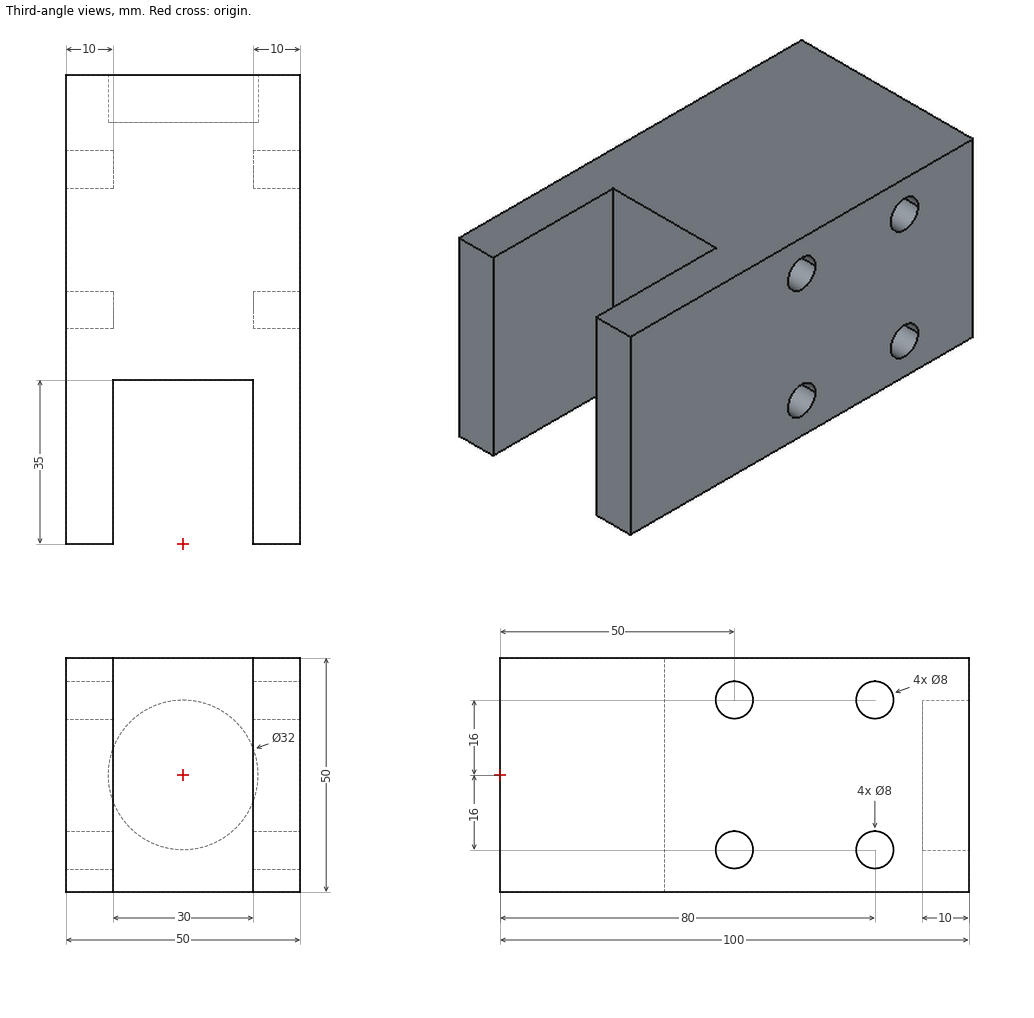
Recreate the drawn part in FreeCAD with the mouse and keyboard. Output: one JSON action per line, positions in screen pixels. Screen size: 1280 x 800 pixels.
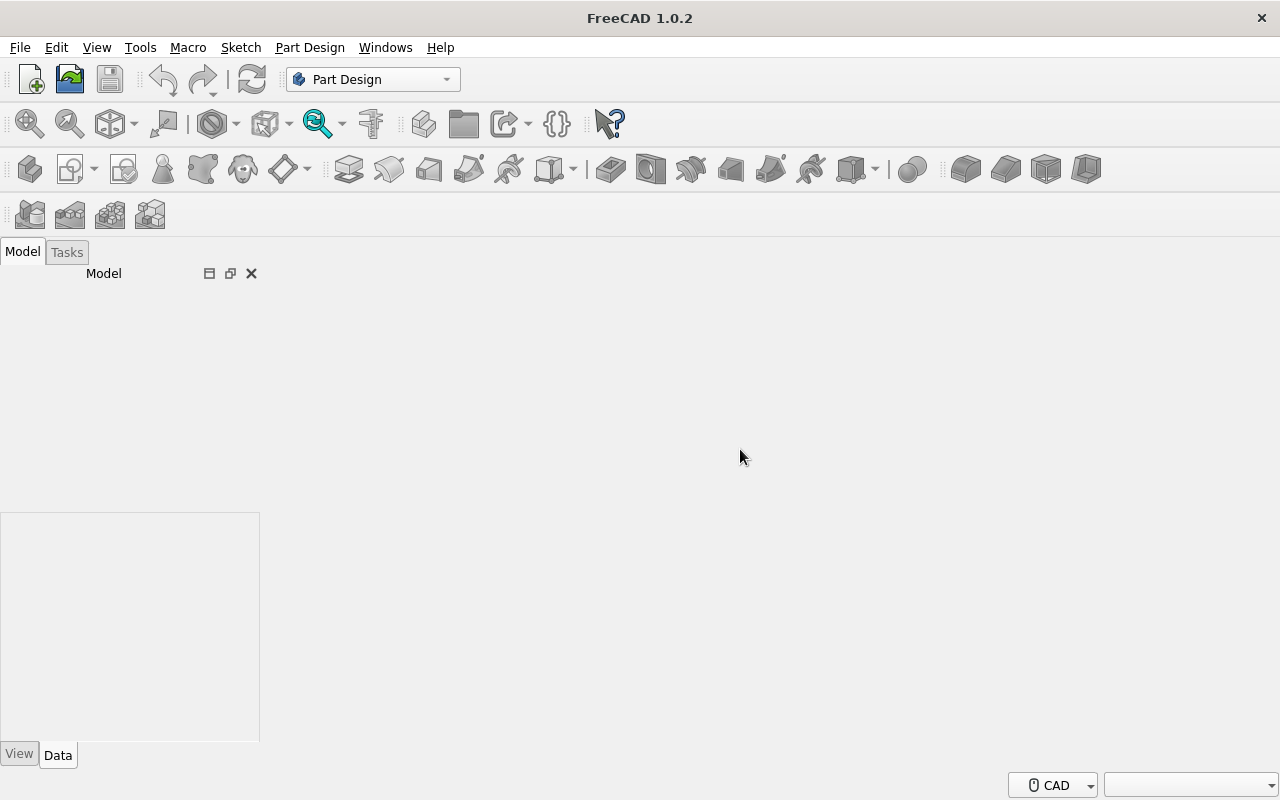
{"action": "left_click", "coordinate": [30, 80]}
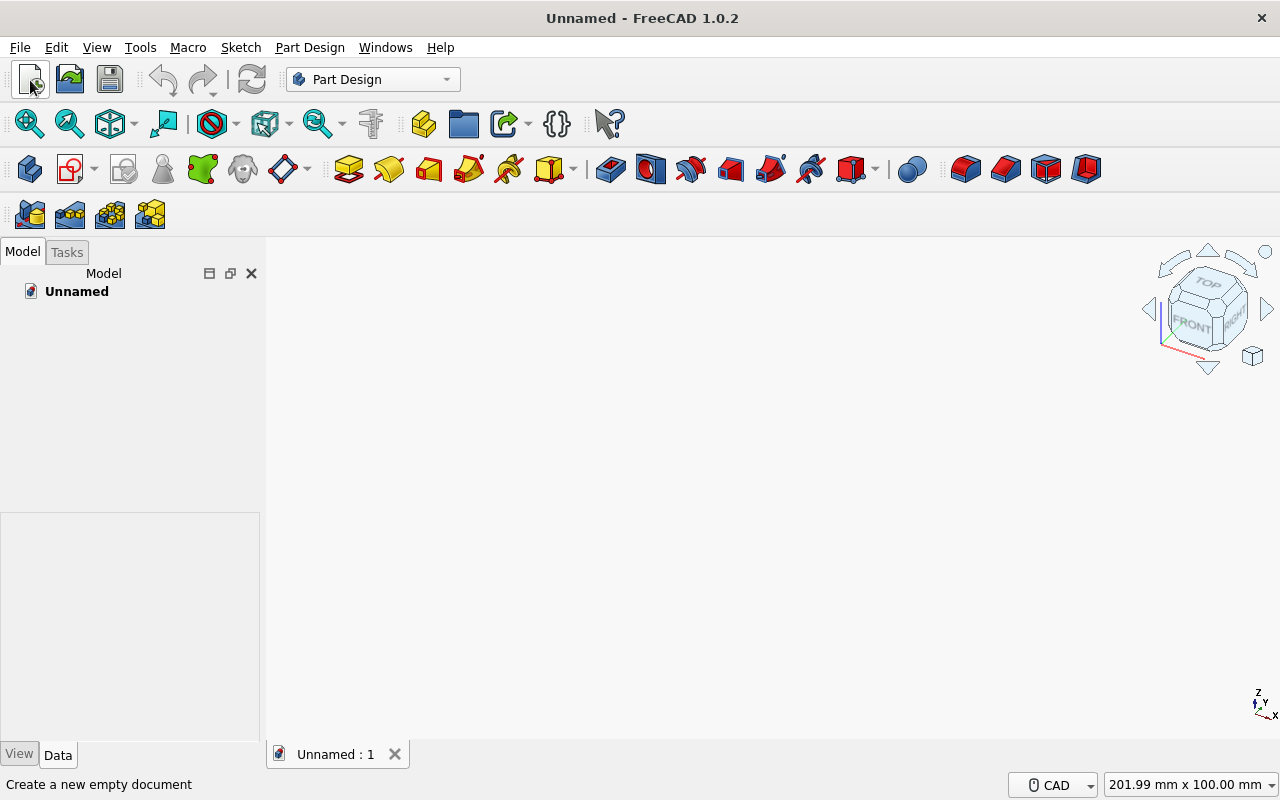
{"action": "left_click", "coordinate": [70, 170]}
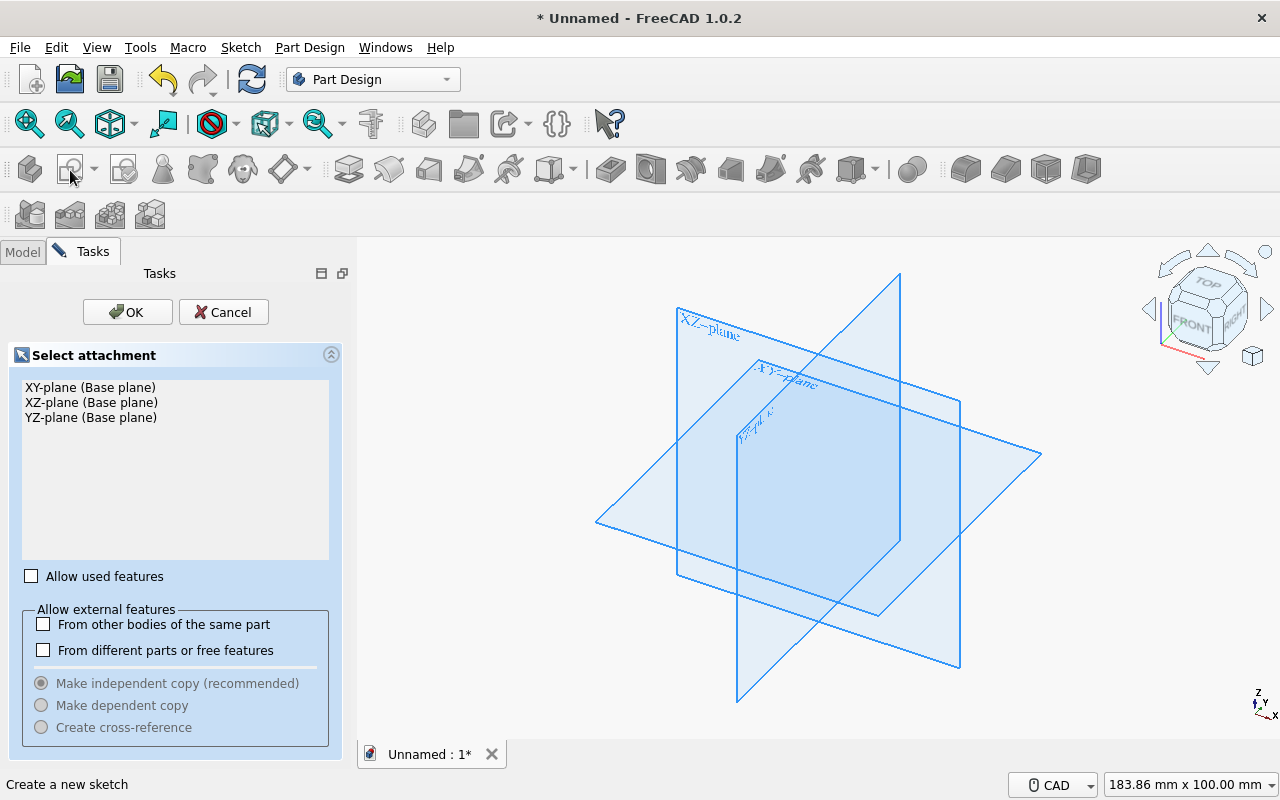
{"action": "left_click", "coordinate": [82, 402]}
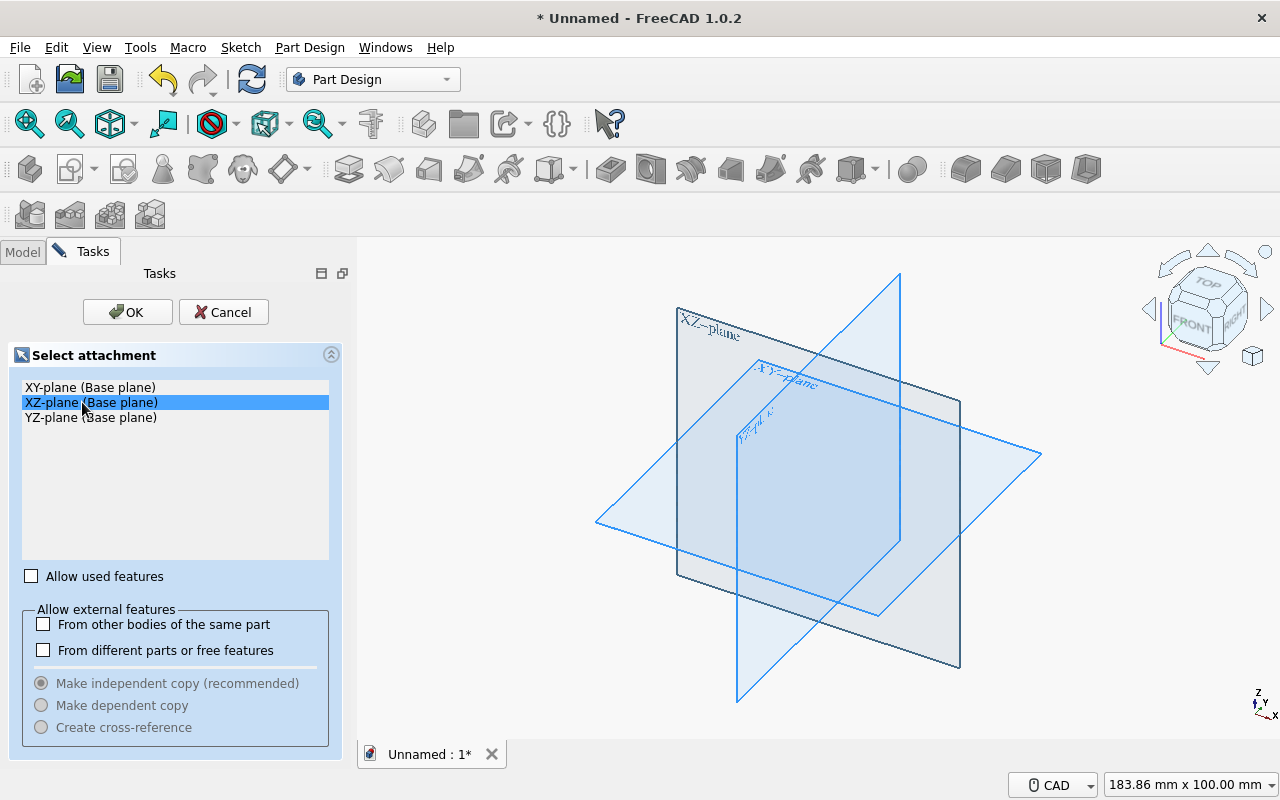
{"action": "left_click", "coordinate": [128, 312]}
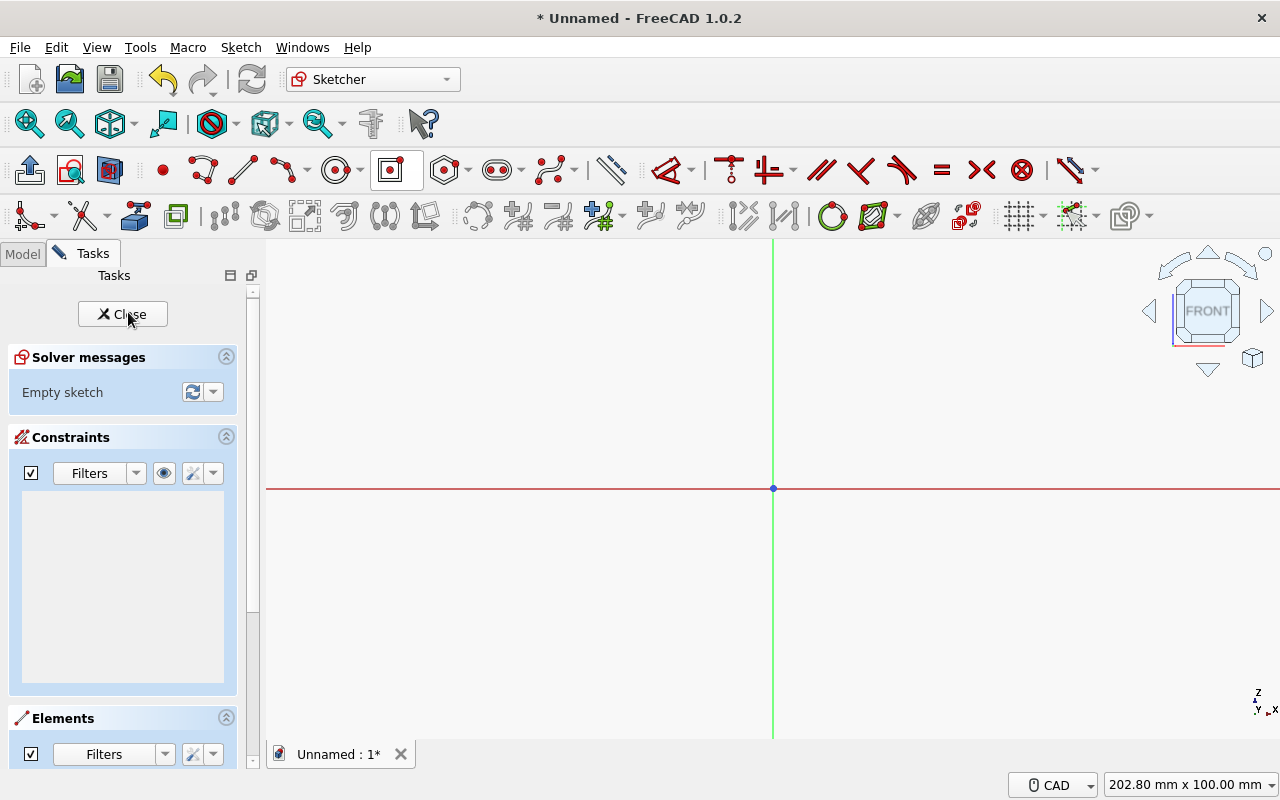
{"action": "left_click", "coordinate": [390, 170]}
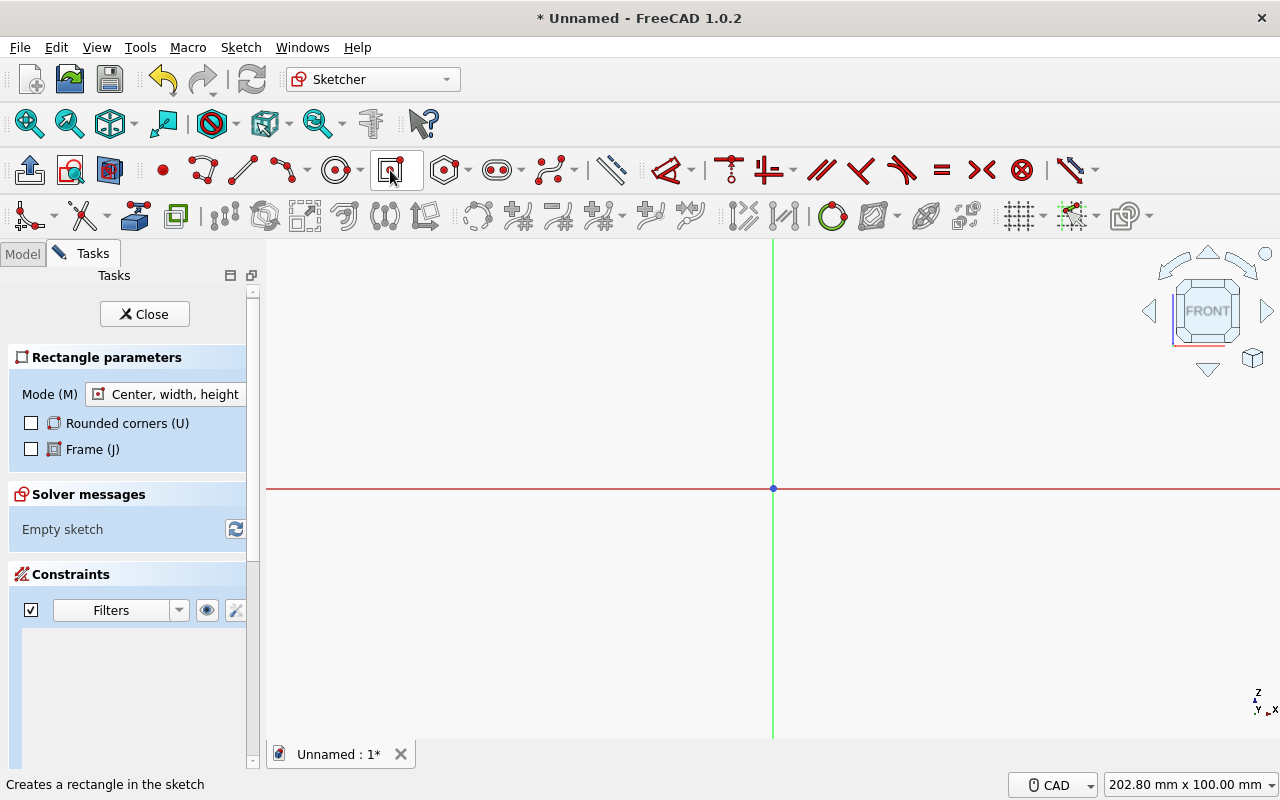
{"action": "left_click", "coordinate": [773, 489]}
{"action": "mouse_move", "coordinate": [898, 364]}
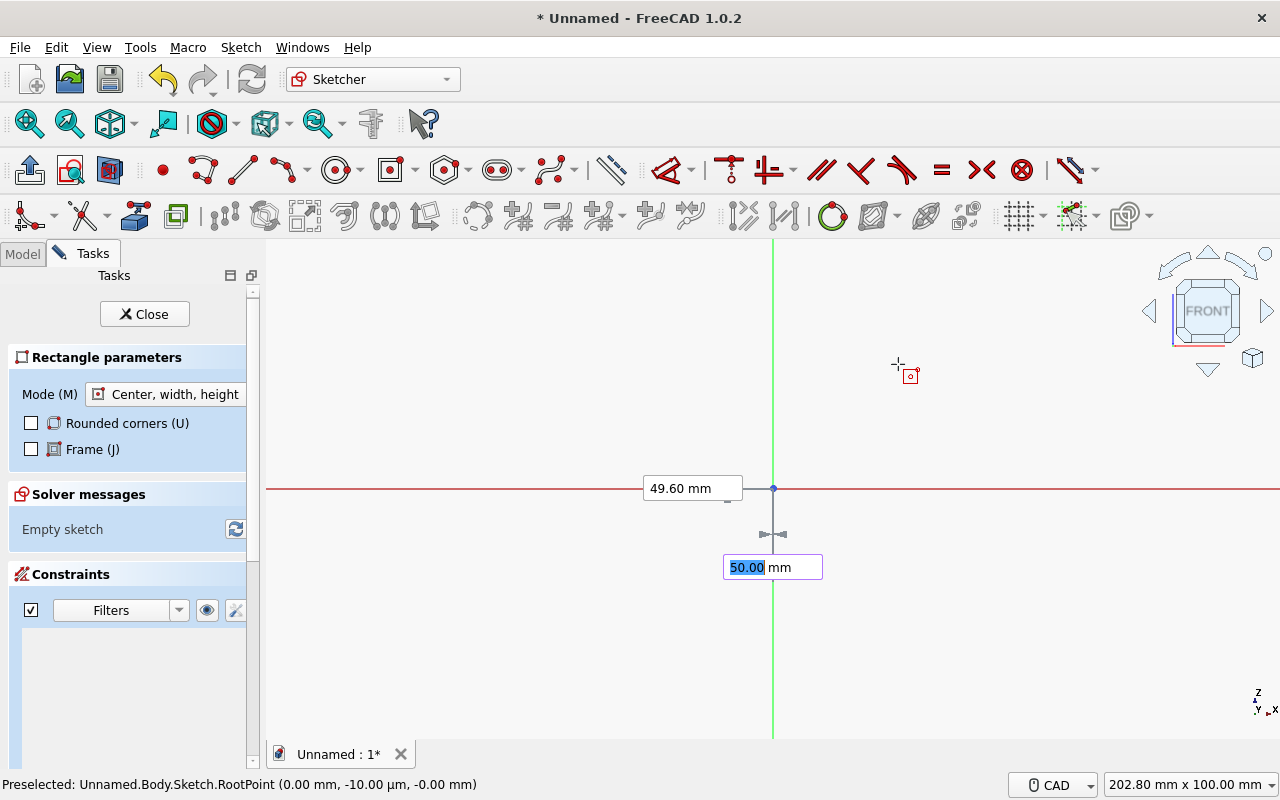
{"action": "type", "text": "50"}
{"action": "key", "text": "Tab"}
{"action": "type", "text": "50"}
{"action": "key", "text": "Return"}
{"action": "key", "text": "Escape"}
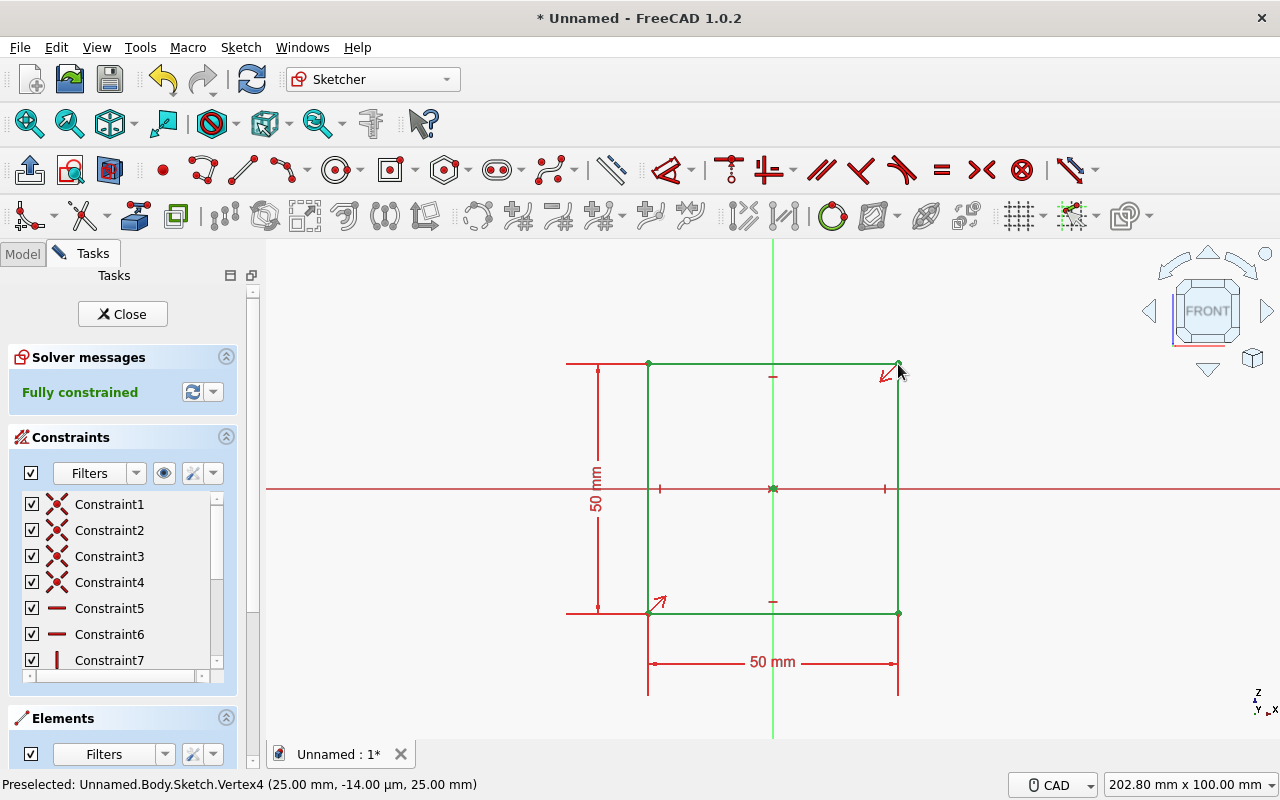
{"action": "left_click", "coordinate": [123, 314]}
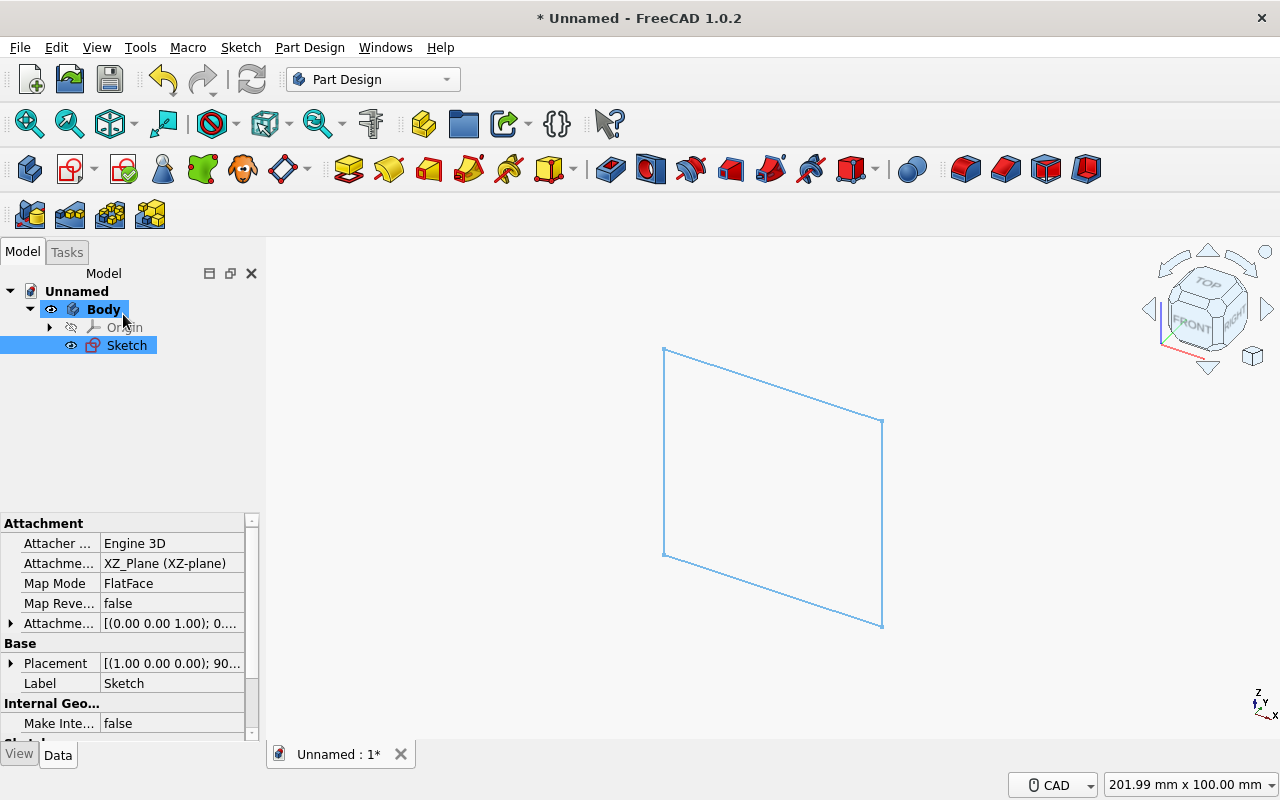
{"action": "left_click", "coordinate": [350, 170]}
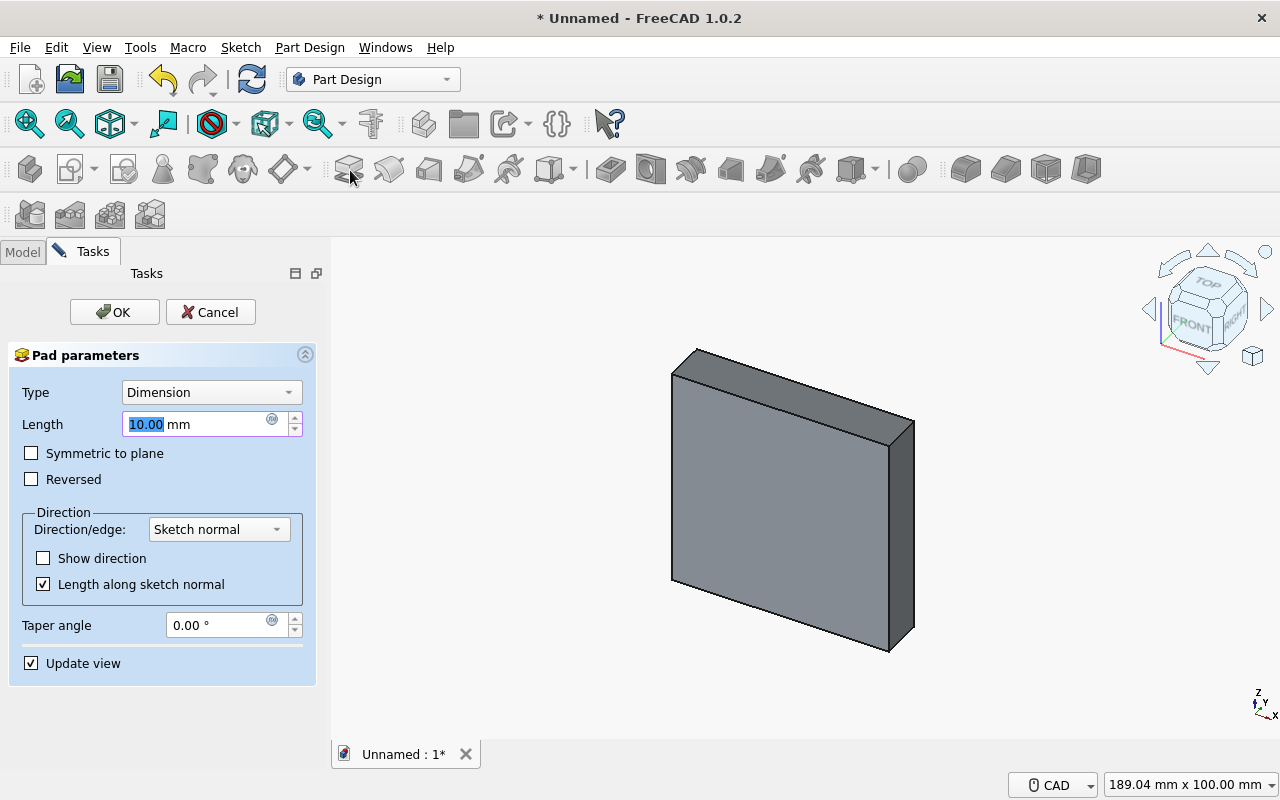
{"action": "type", "text": "100"}
{"action": "key", "text": "Tab"}